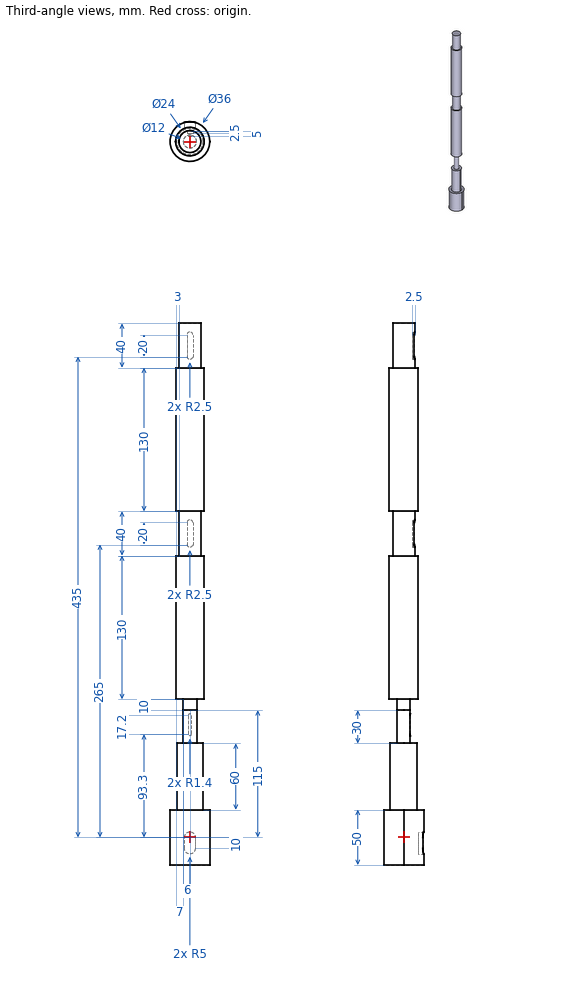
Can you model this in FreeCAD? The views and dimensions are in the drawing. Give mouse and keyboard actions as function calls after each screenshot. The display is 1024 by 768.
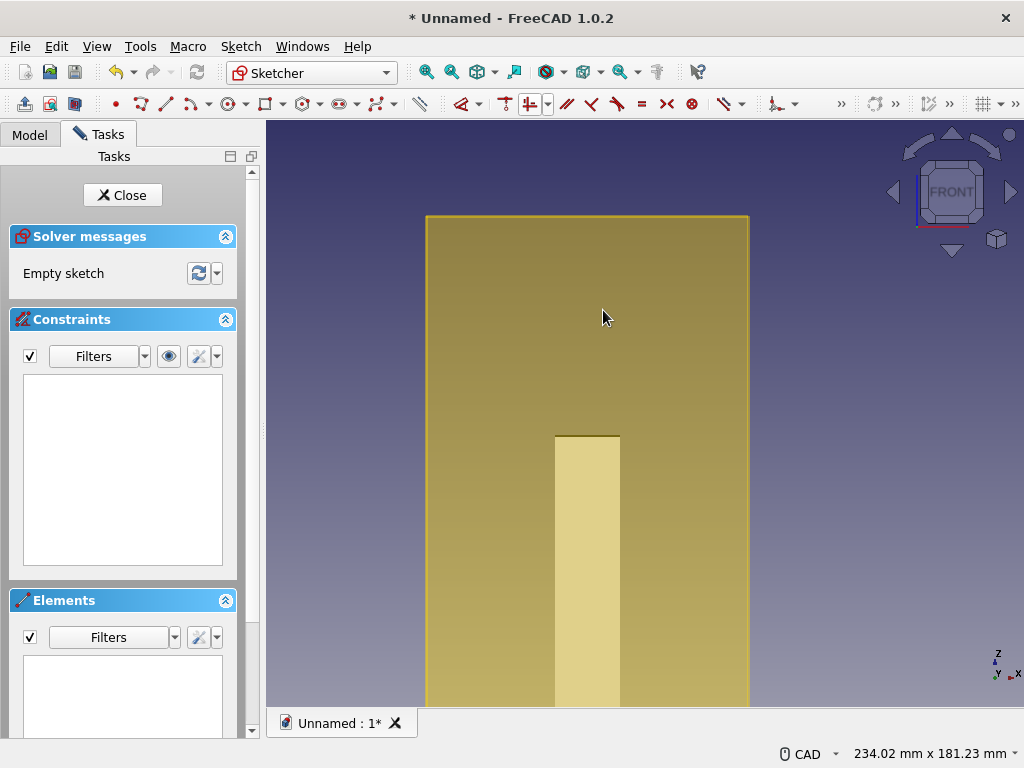
scroll(556, 415, up, 3)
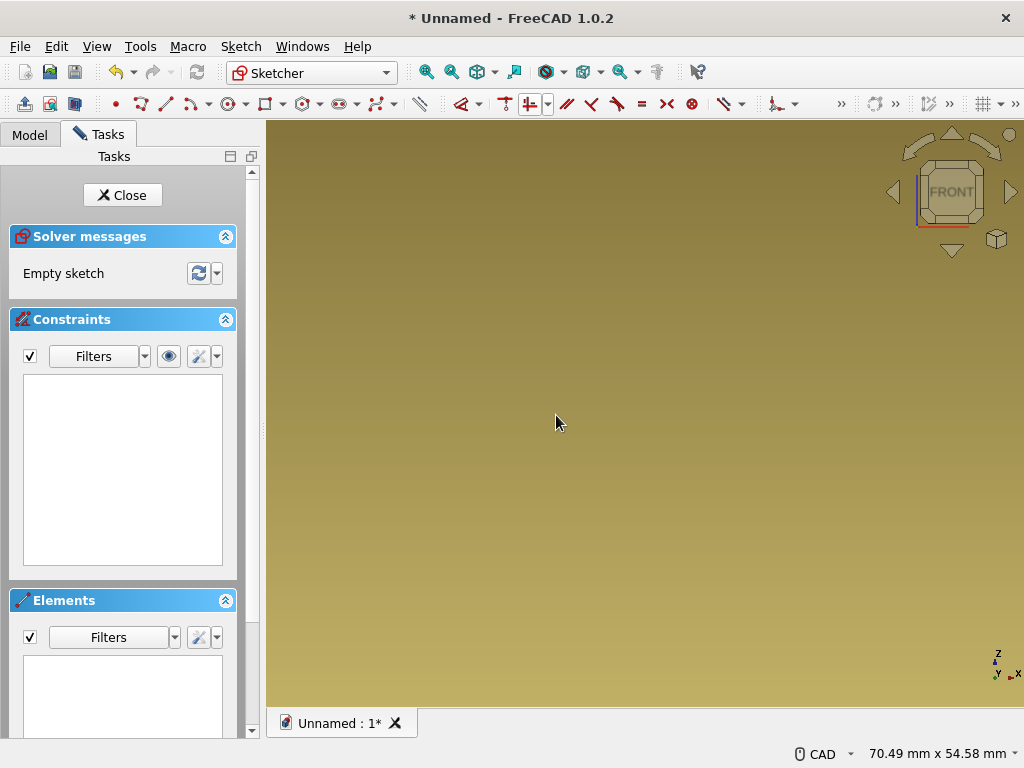
click(338, 104)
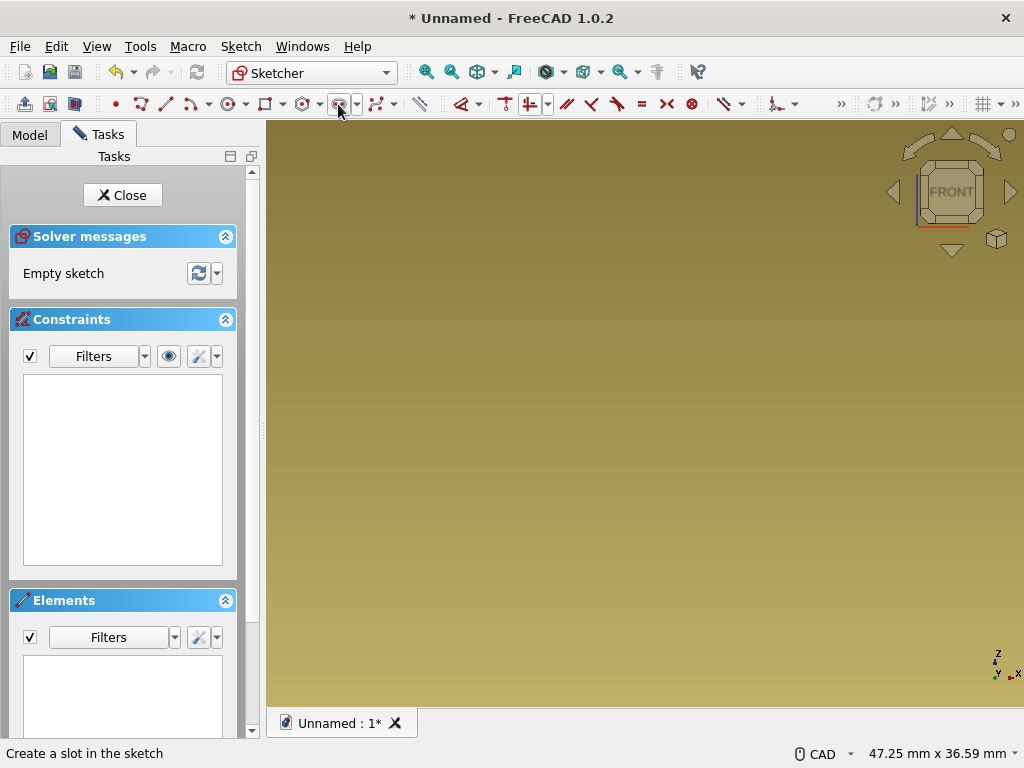
click(576, 574)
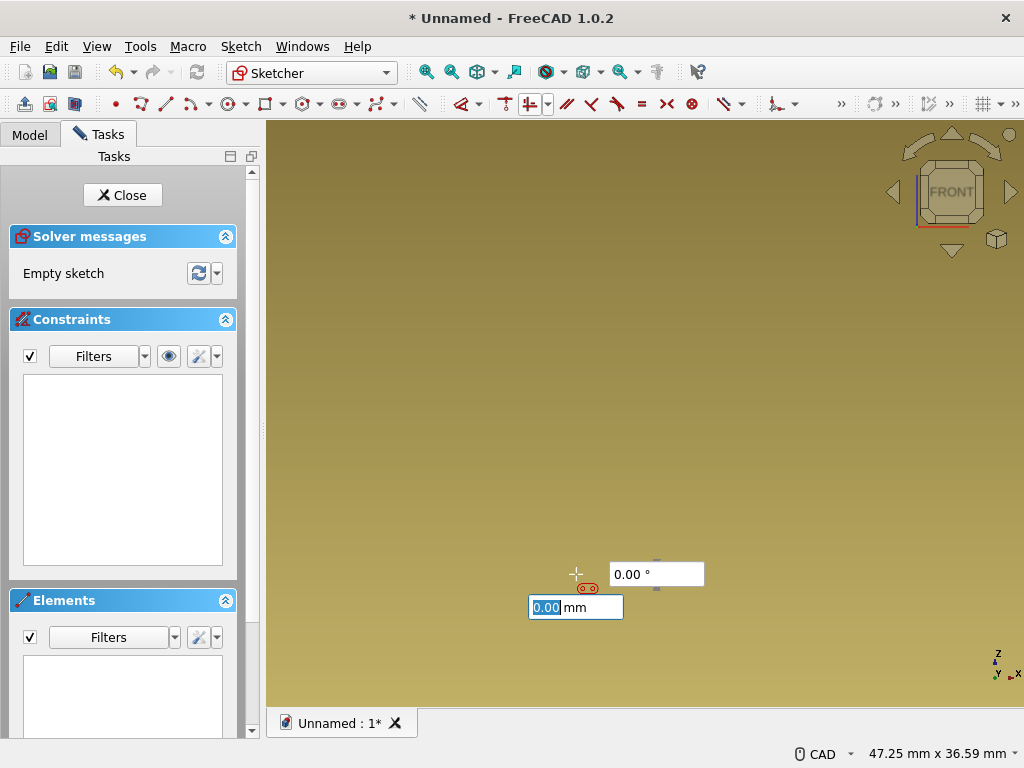
click(585, 253)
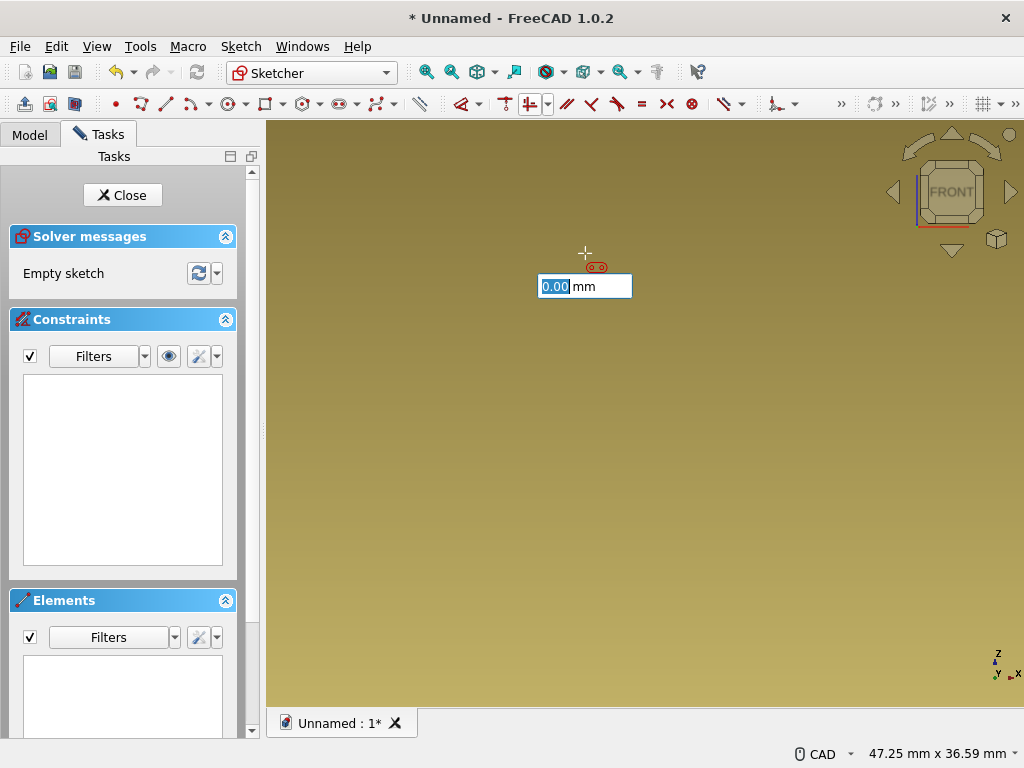
click(616, 413)
key(Escape)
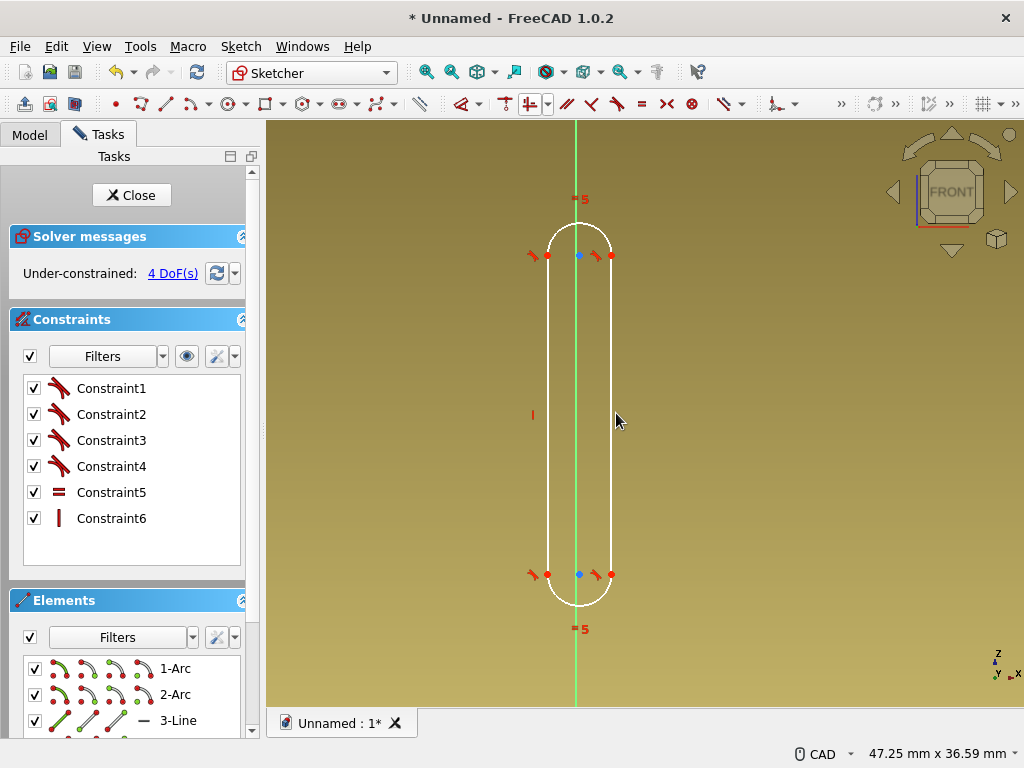
click(580, 574)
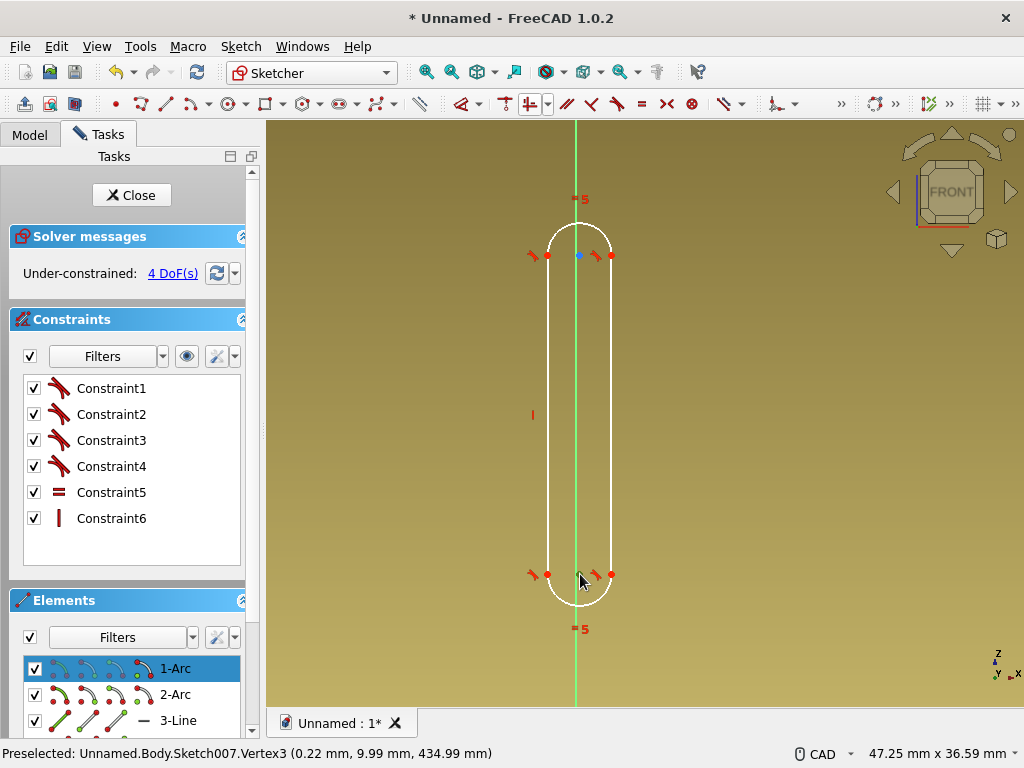
click(576, 641)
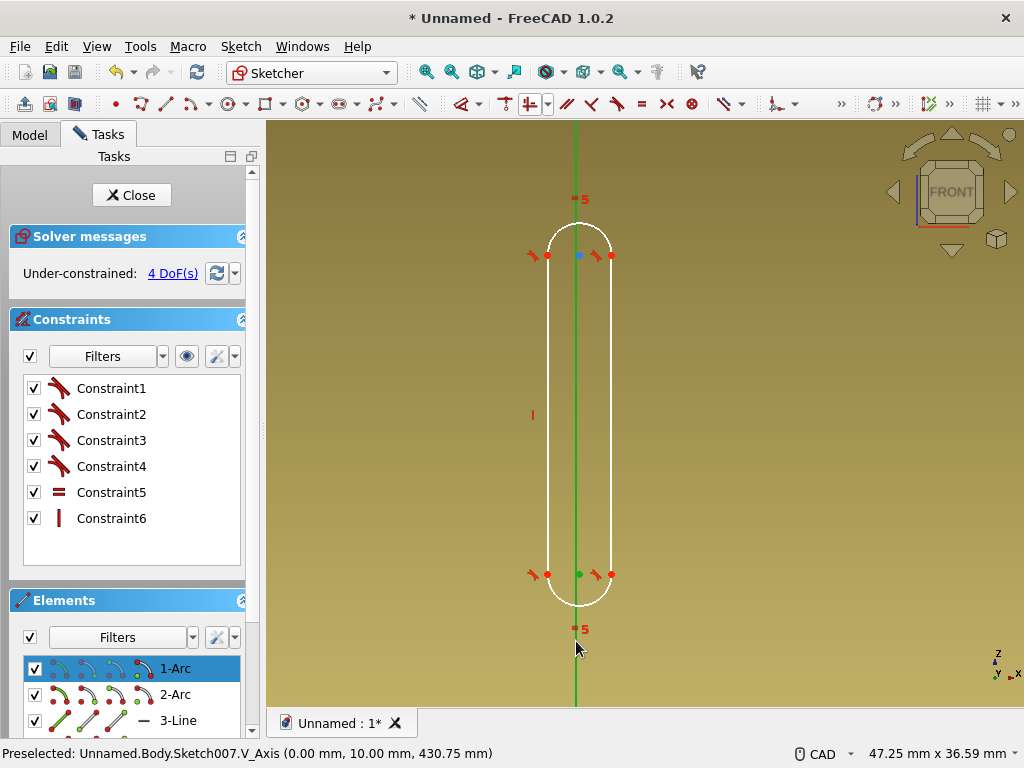
click(505, 104)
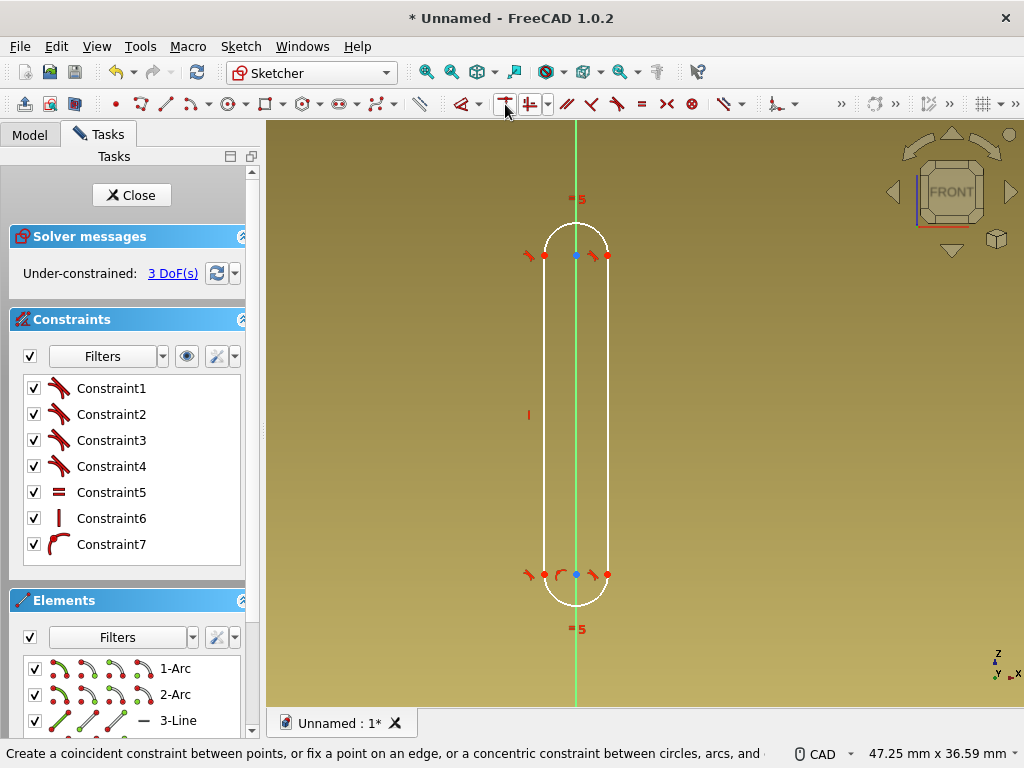
click(460, 104)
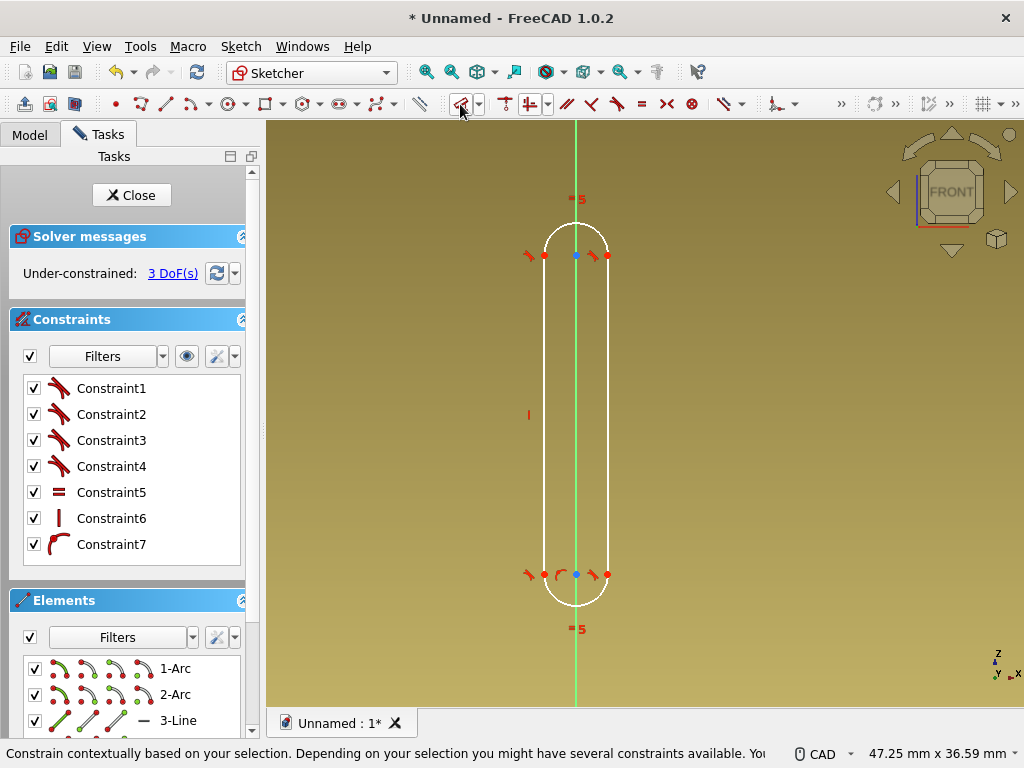
click(557, 600)
click(538, 626)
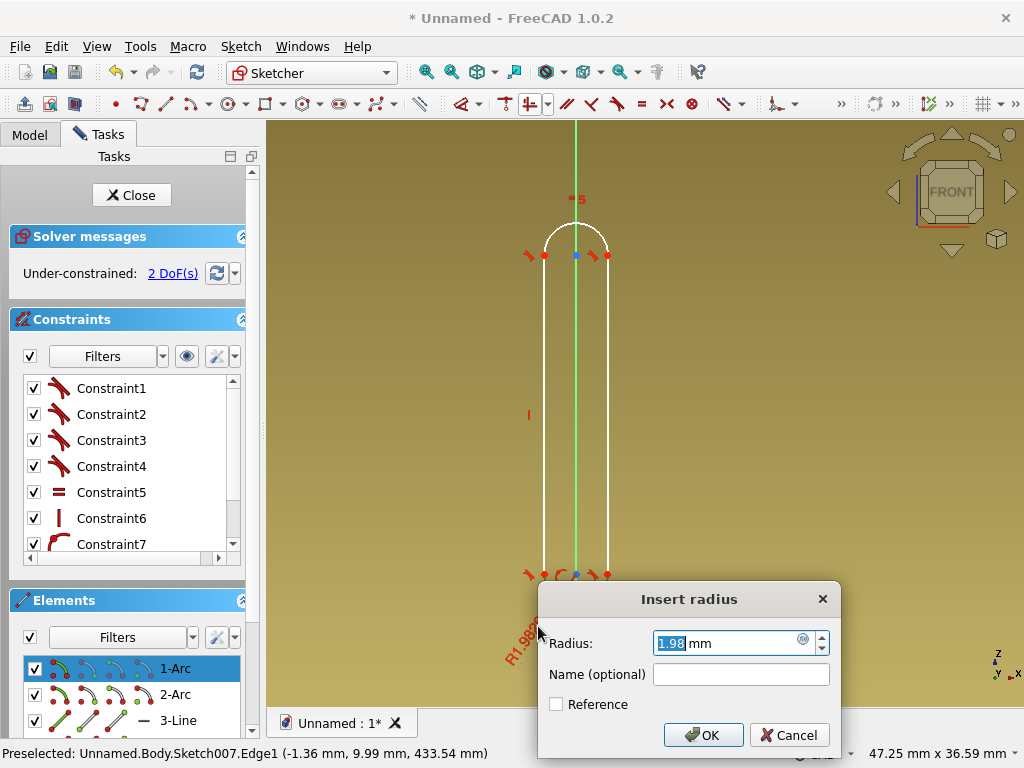
text(2.5)
key(Return)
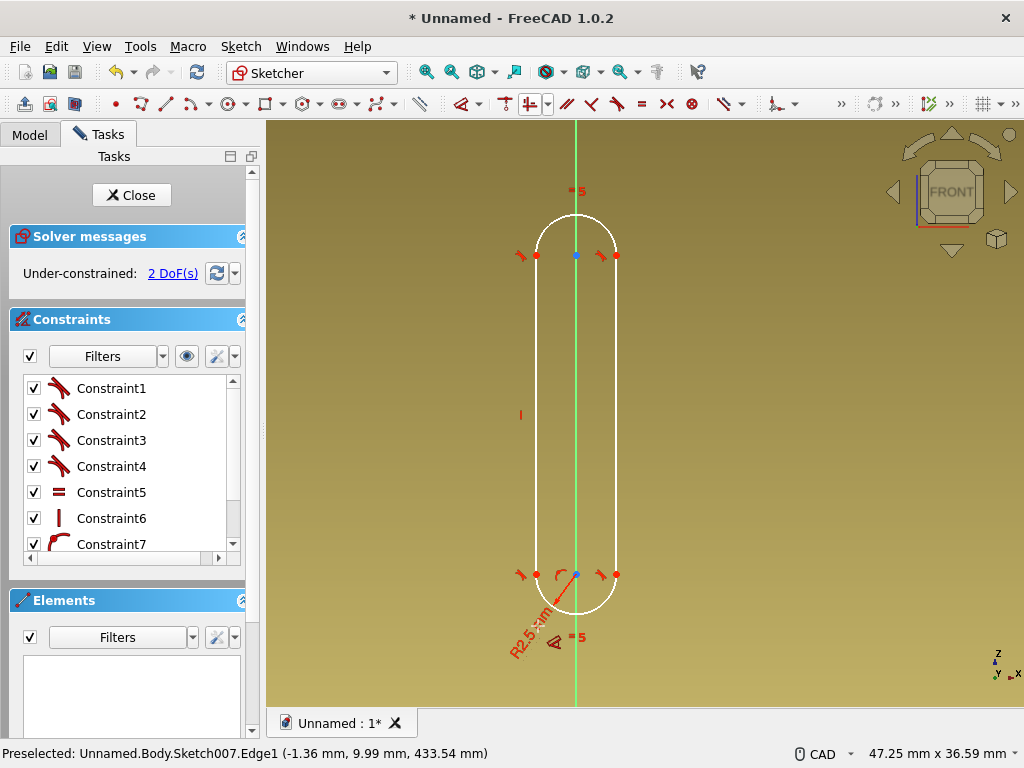
click(536, 478)
click(502, 415)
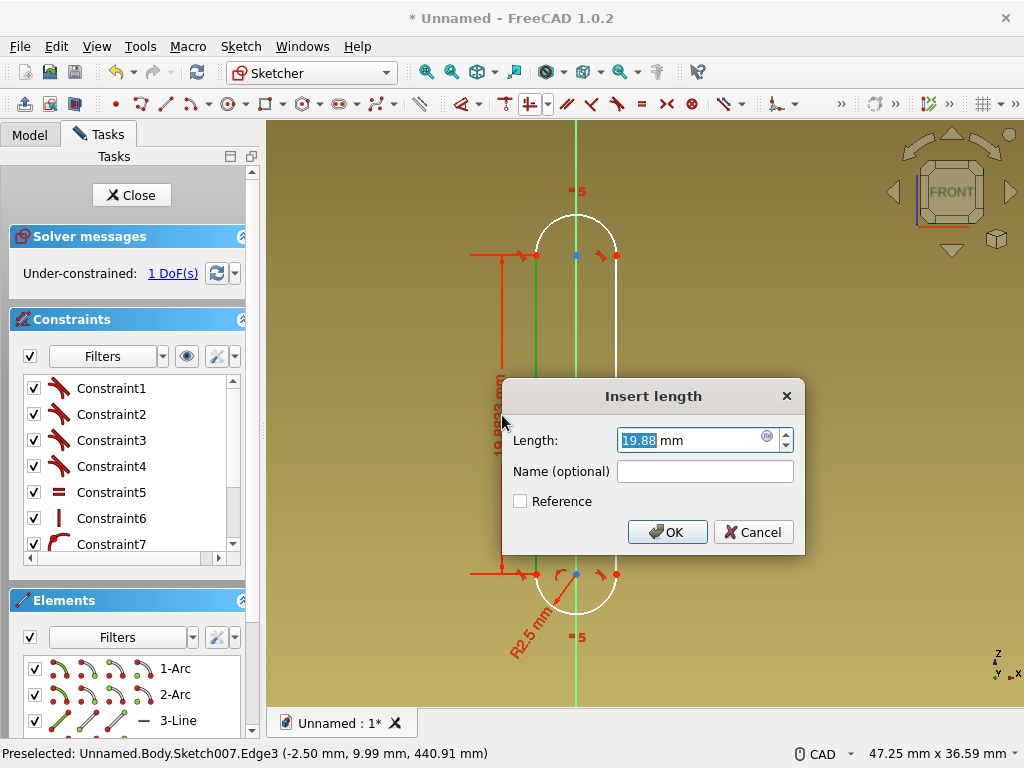
text(20)
key(Return)